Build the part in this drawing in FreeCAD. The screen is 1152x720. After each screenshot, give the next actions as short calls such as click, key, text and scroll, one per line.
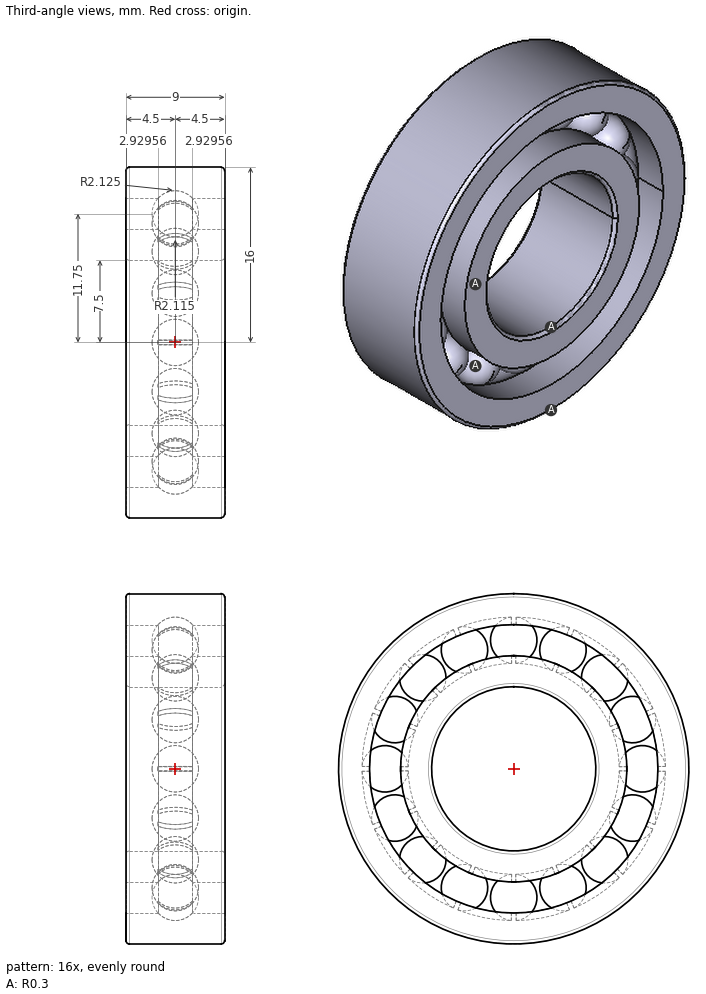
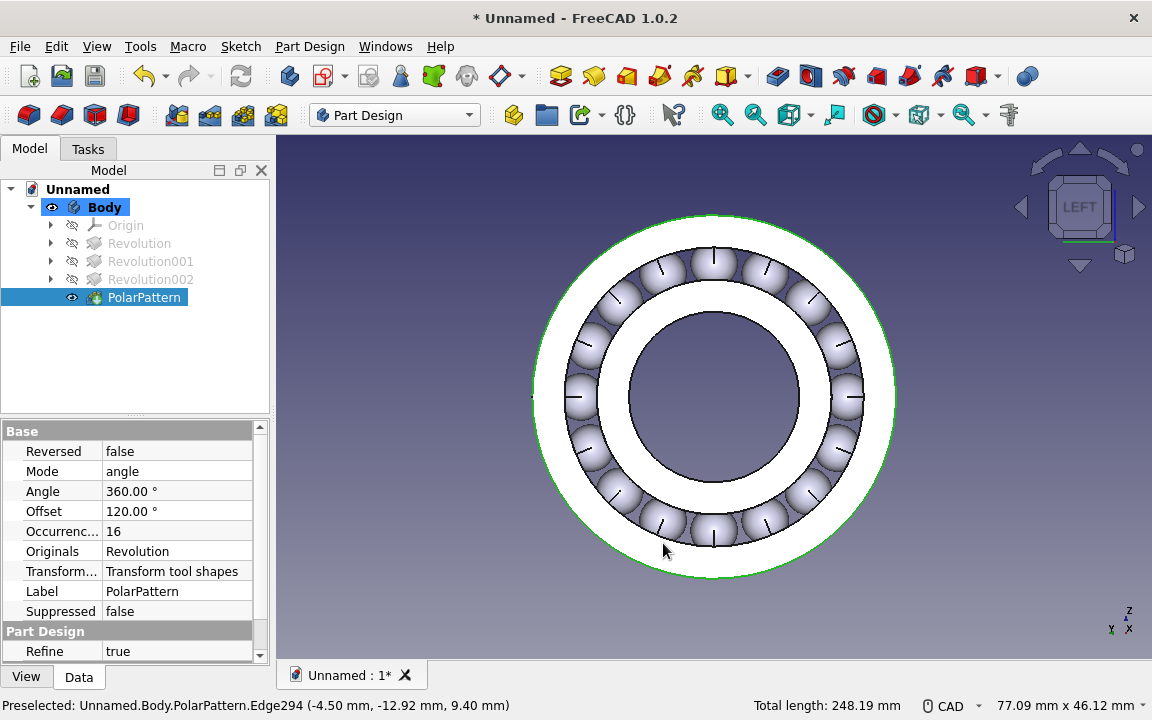
click(799, 396, ctrl)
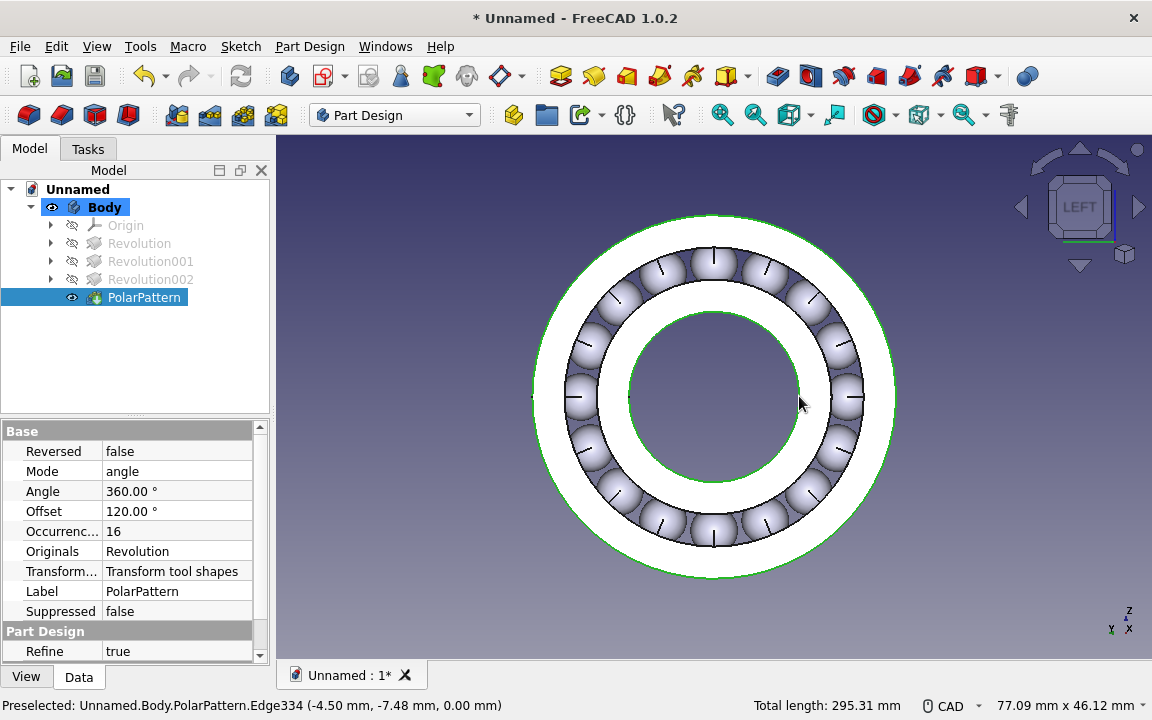
click(29, 116)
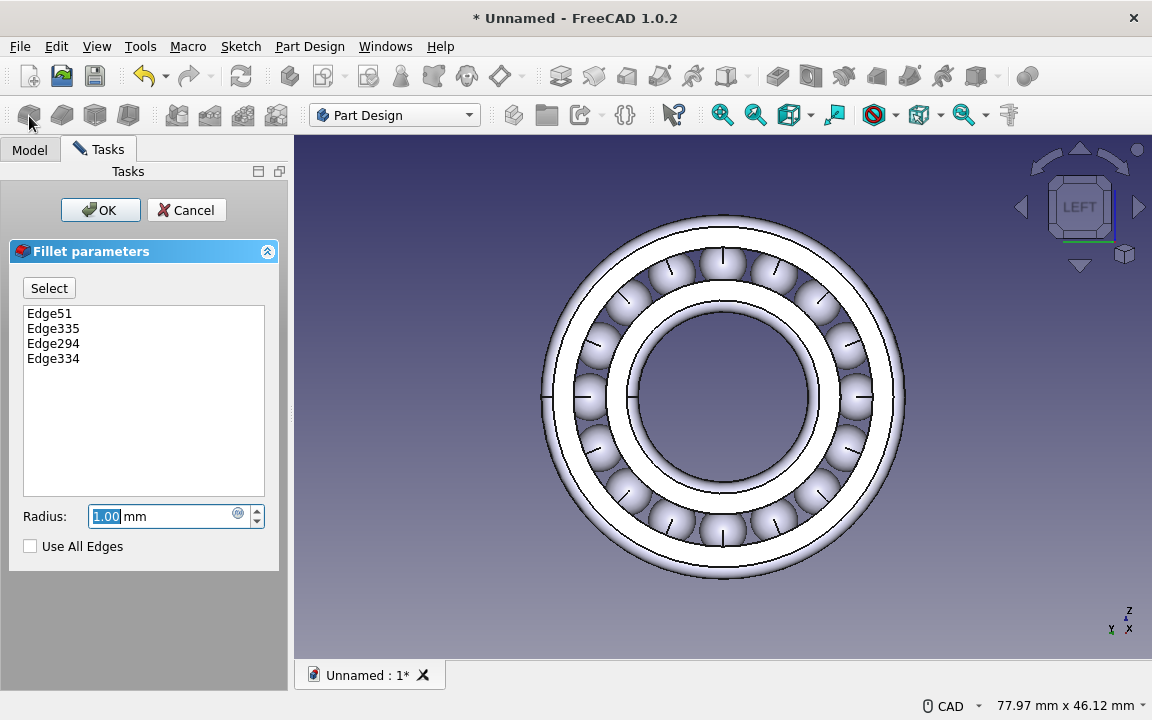
text(0.3)
key(Tab)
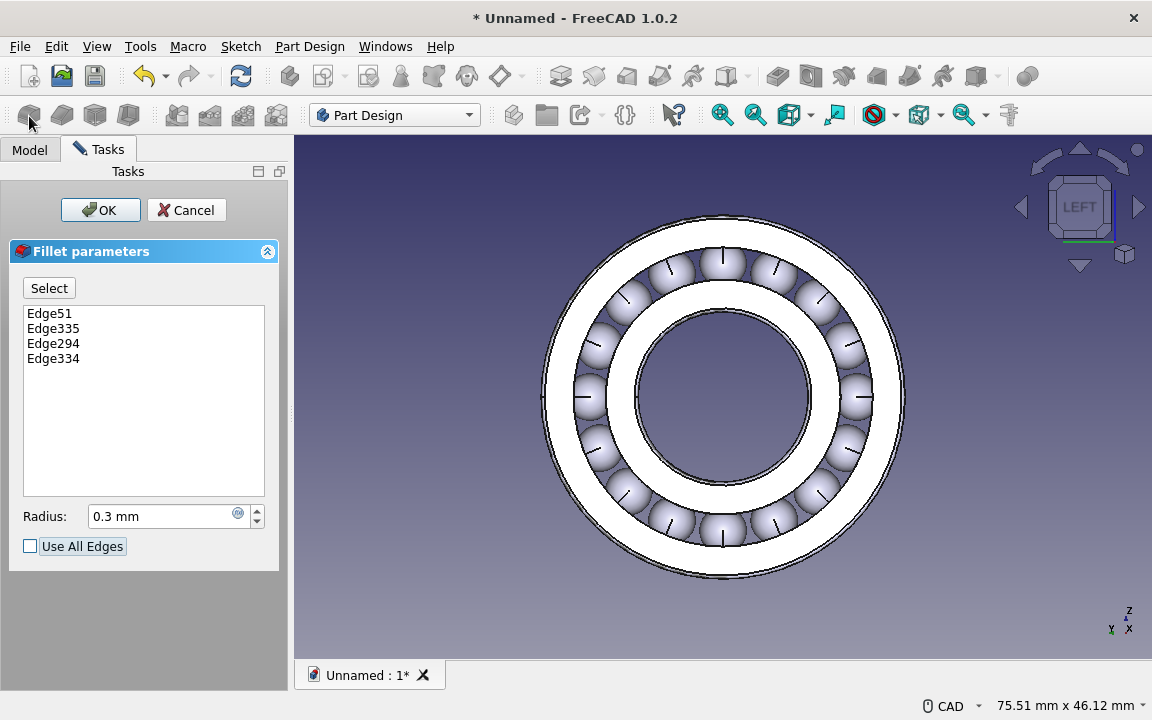
click(101, 210)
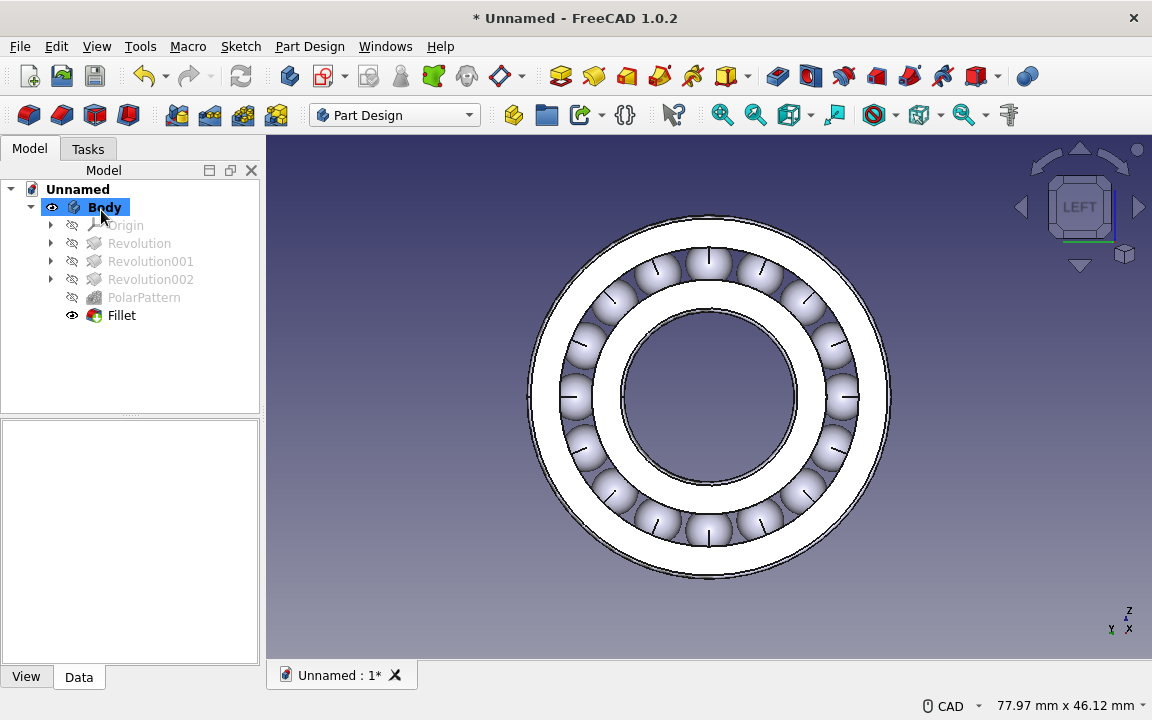
key(0)